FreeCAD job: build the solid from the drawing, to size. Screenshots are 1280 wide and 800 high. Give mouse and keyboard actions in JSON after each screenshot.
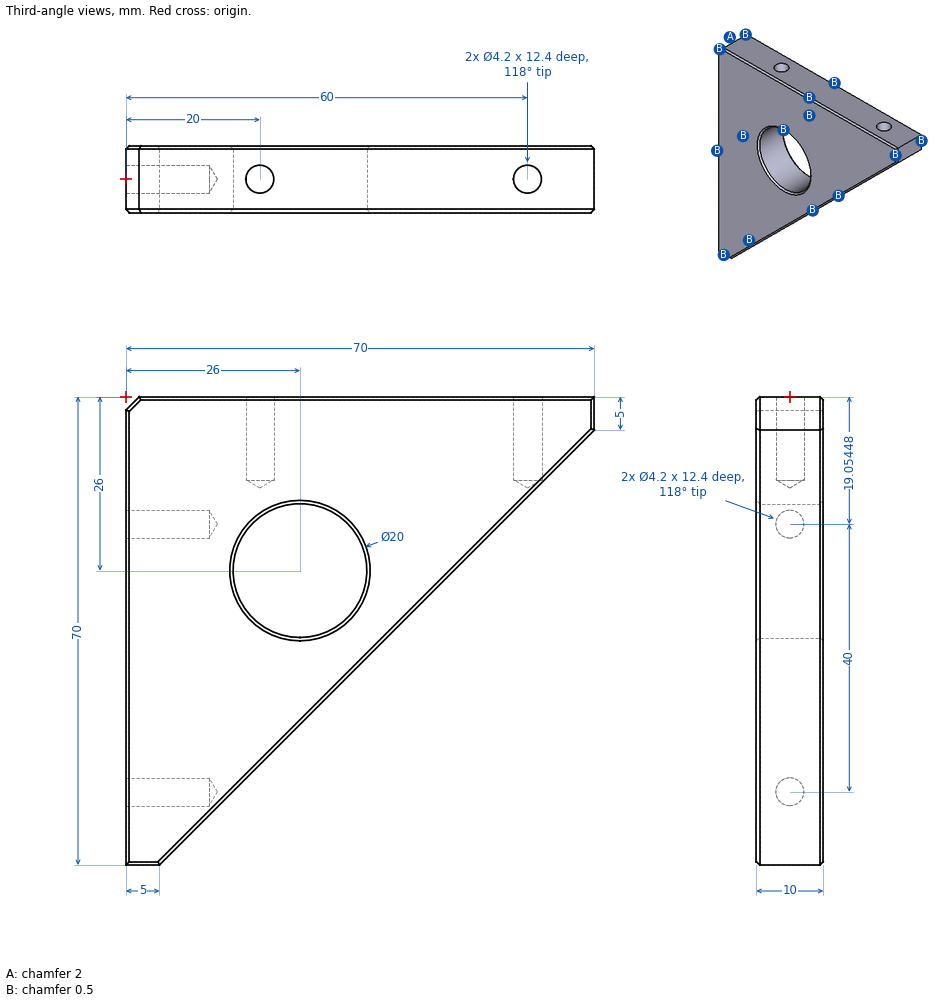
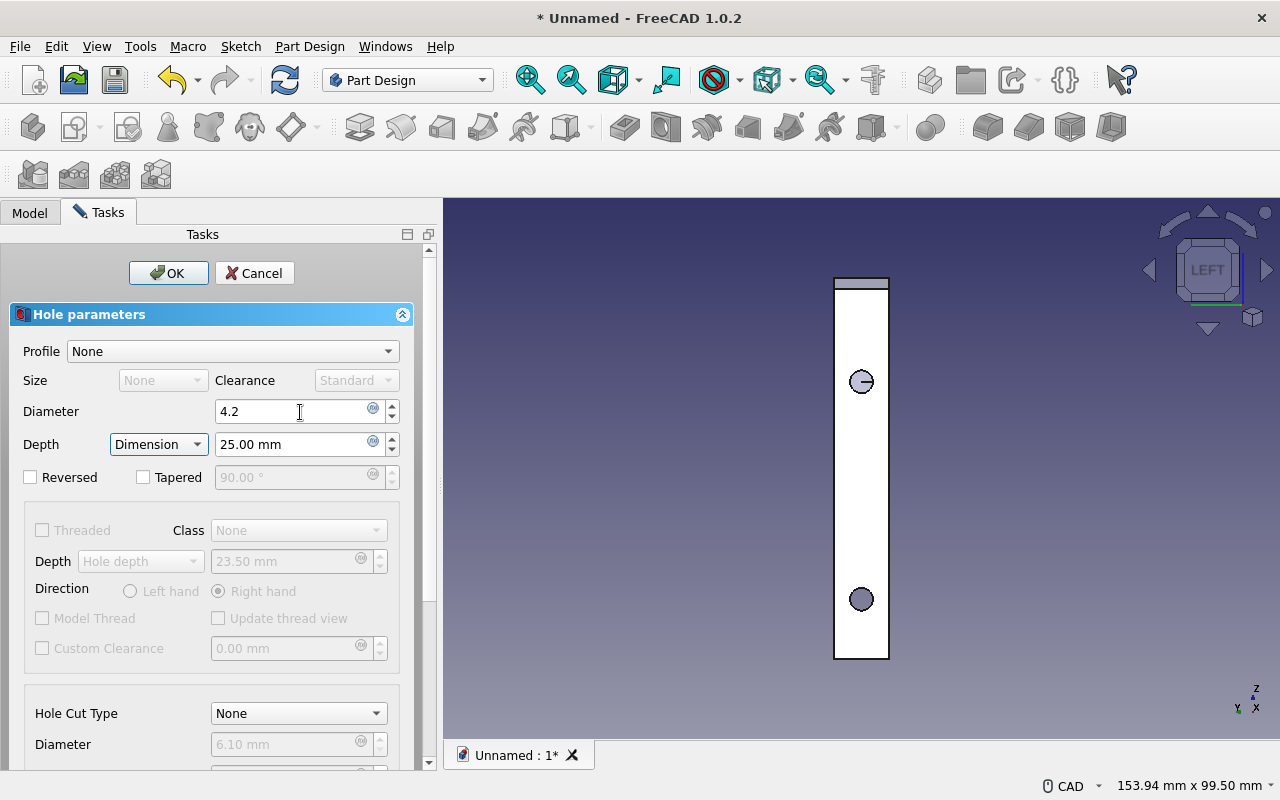
{"action": "triple_click", "coordinate": [300, 444]}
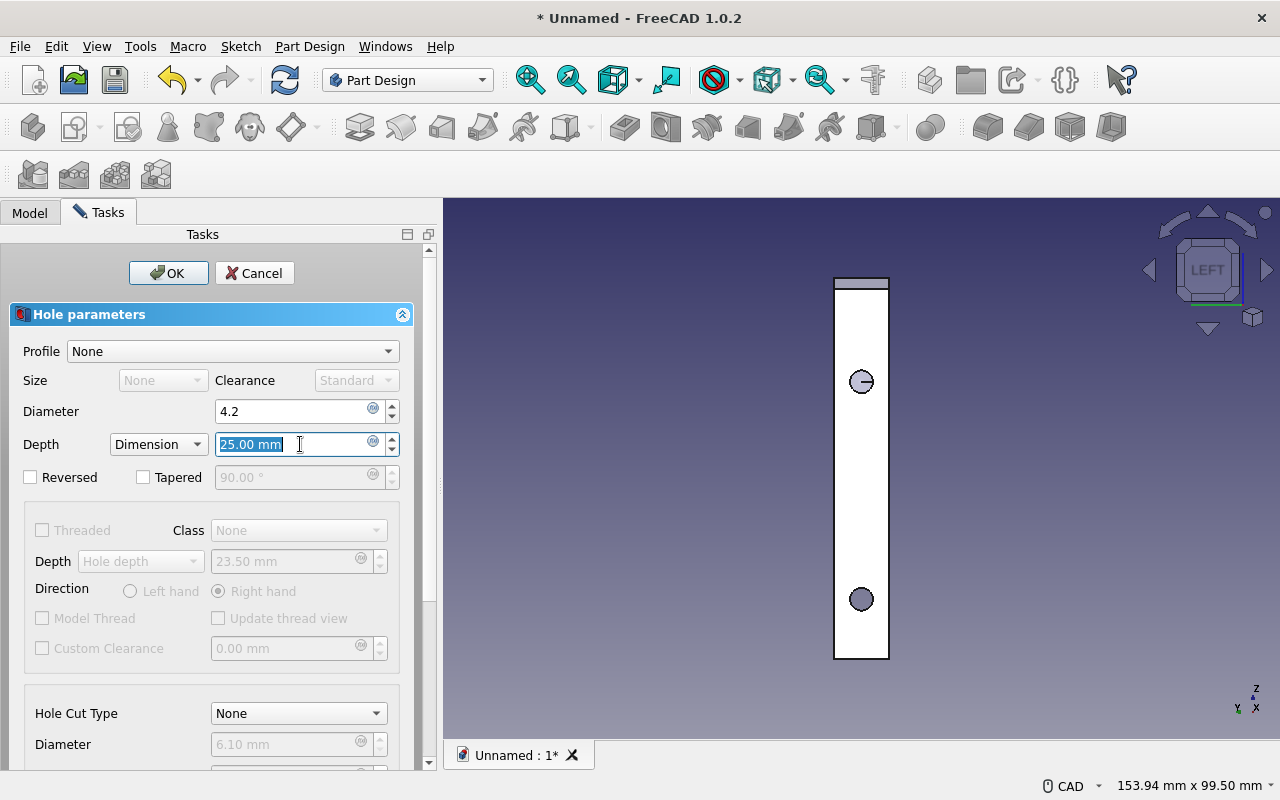
{"action": "type", "text": "12.4"}
{"action": "key", "text": "Tab"}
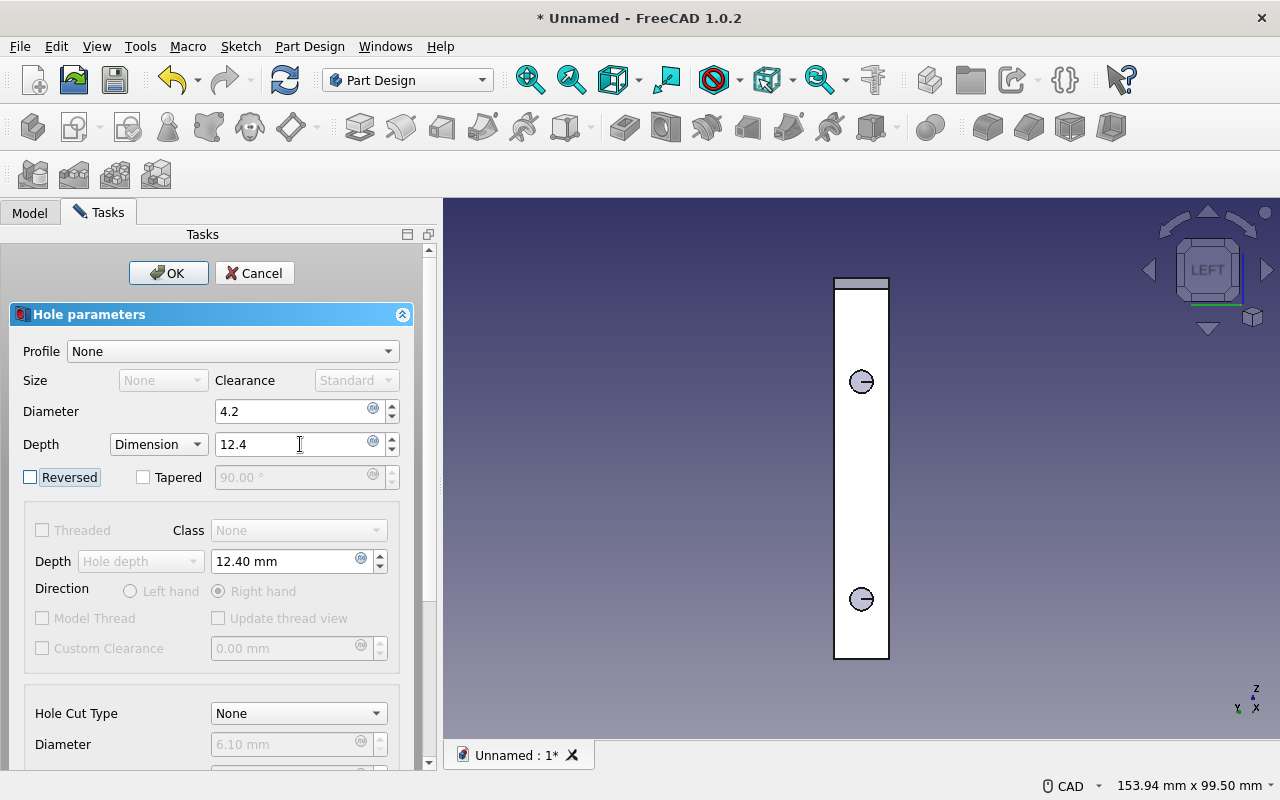
{"action": "left_click", "coordinate": [169, 273]}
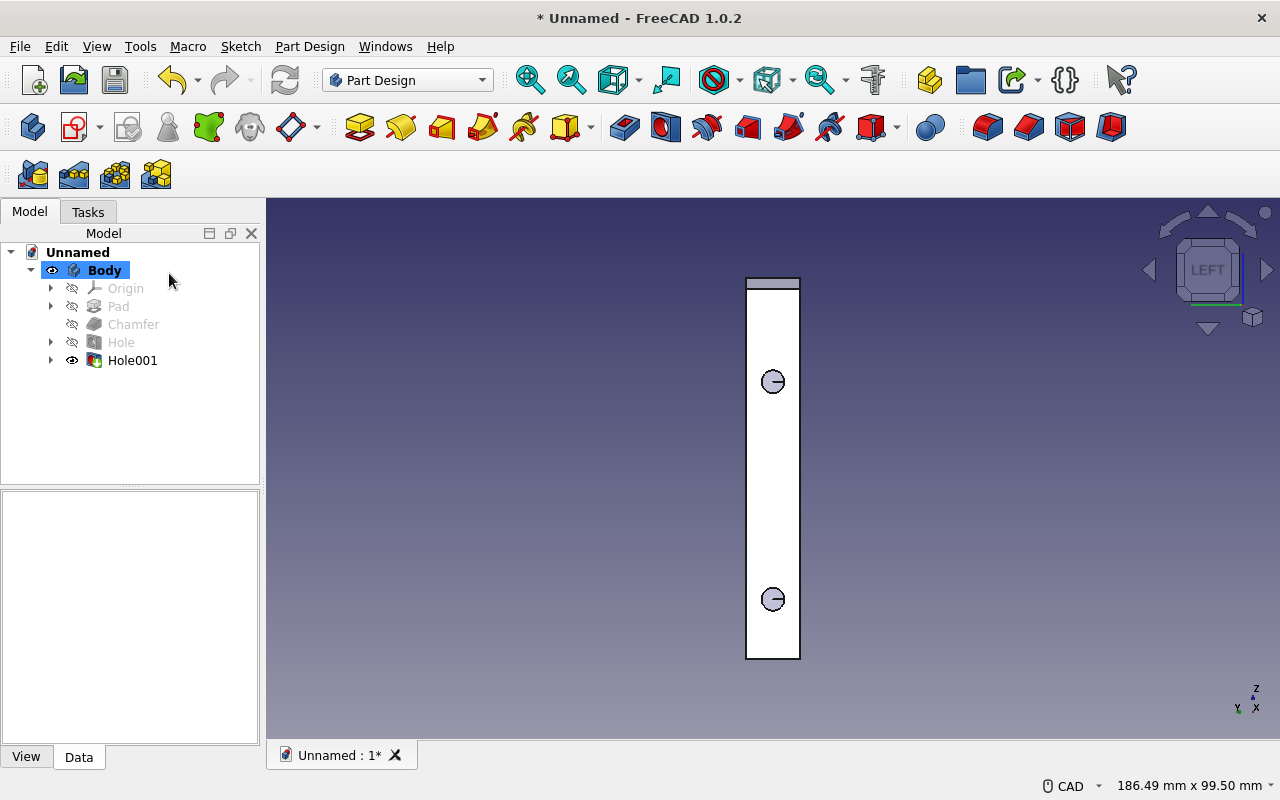
{"action": "key", "text": "0"}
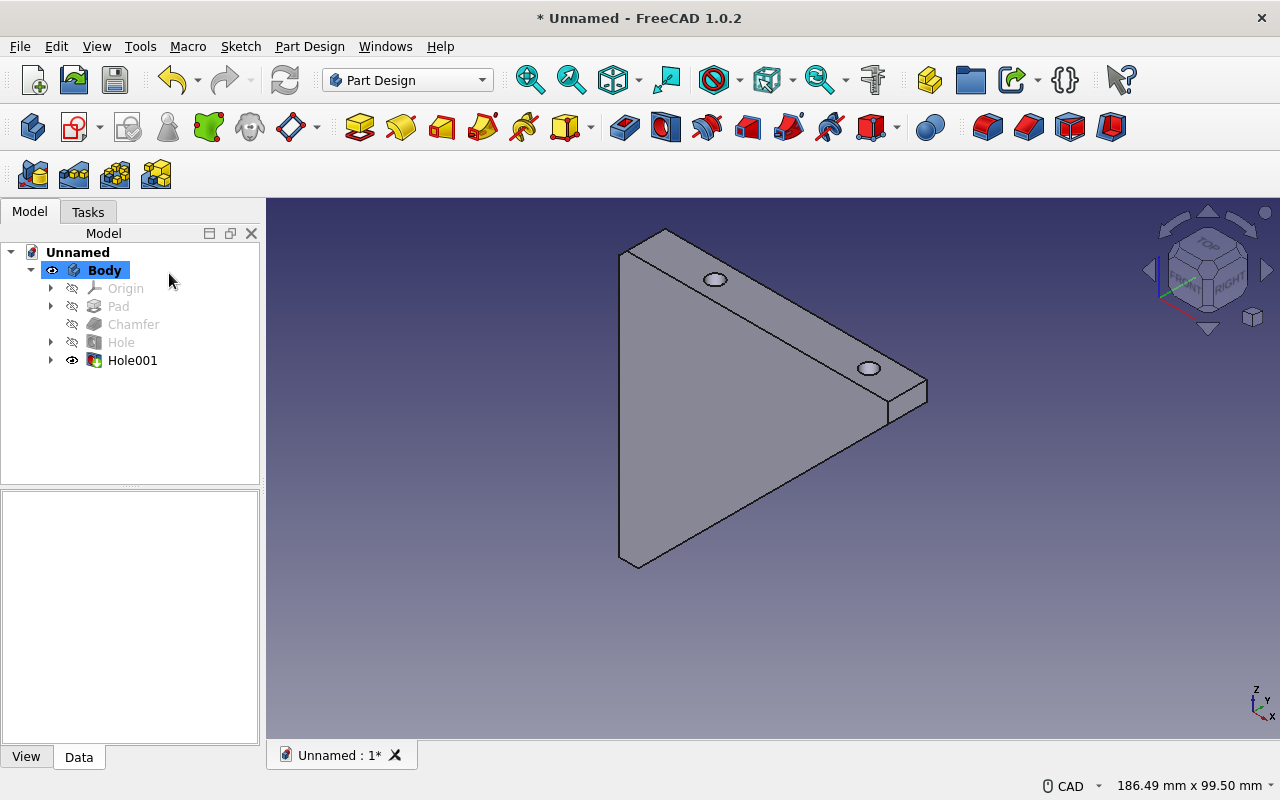
{"action": "left_click", "coordinate": [715, 412]}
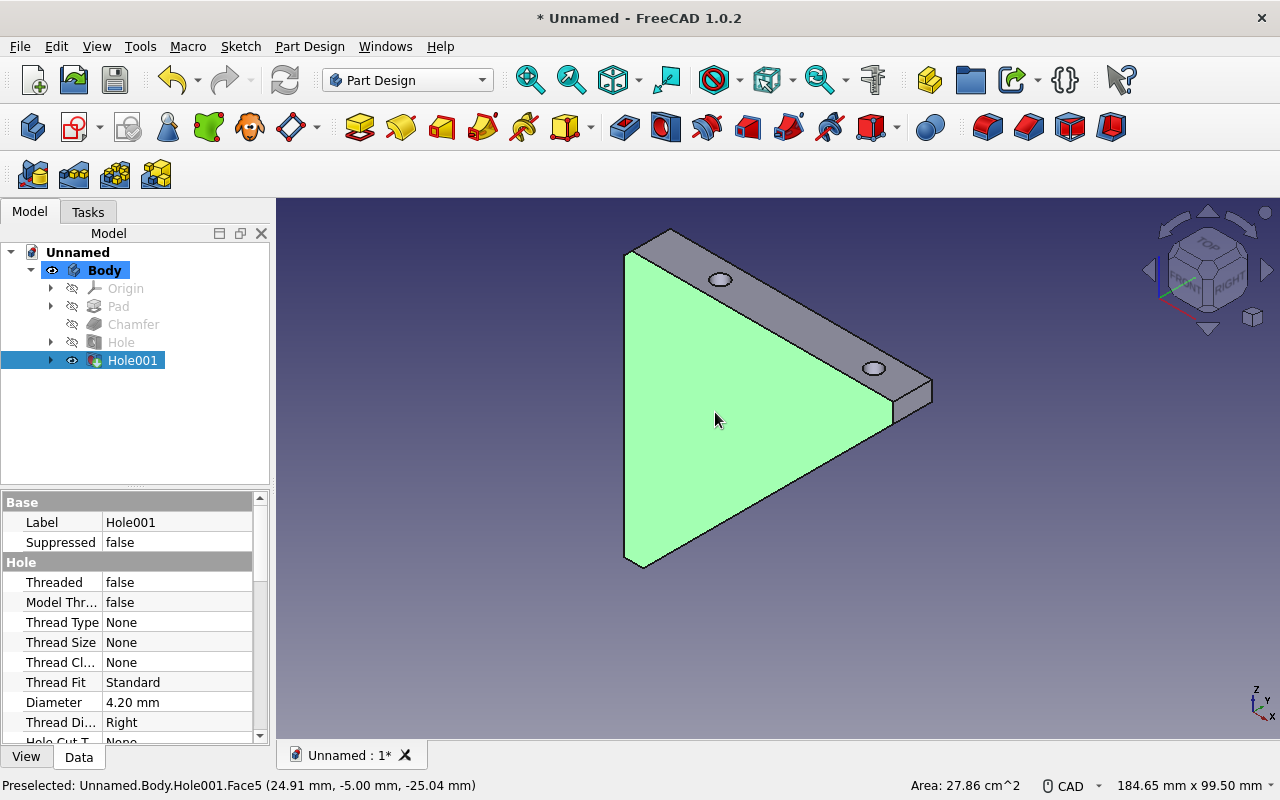
{"action": "left_click", "coordinate": [74, 128]}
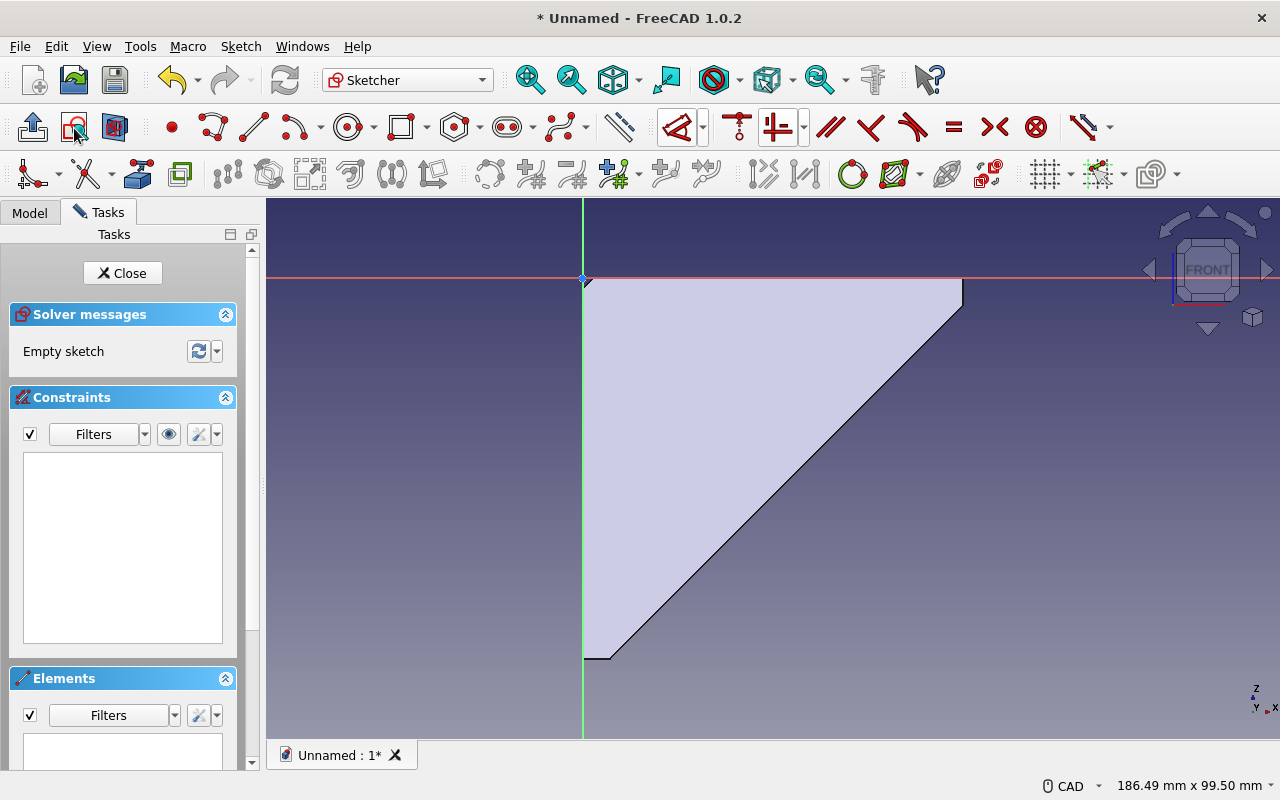
{"action": "scroll", "coordinate": [651, 264], "scroll_direction": "up", "scroll_amount": 3}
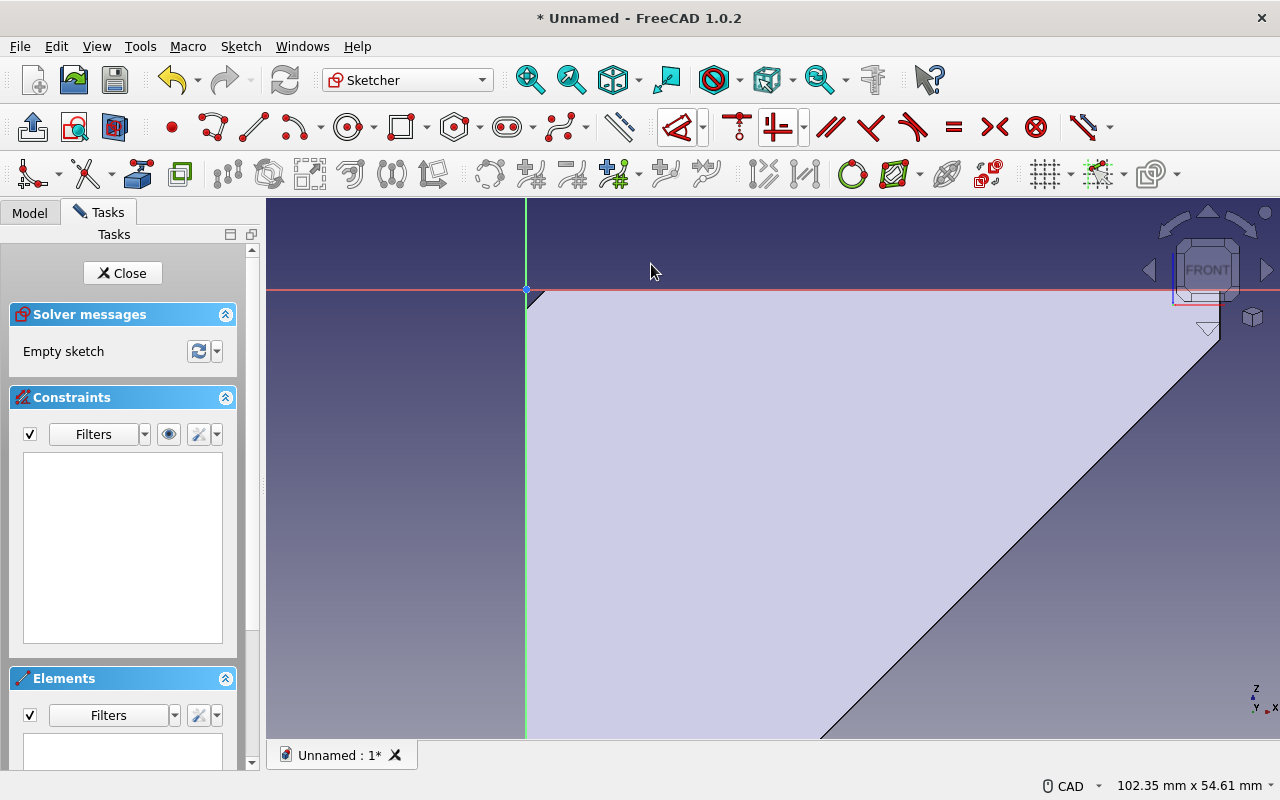
{"action": "left_click", "coordinate": [348, 128]}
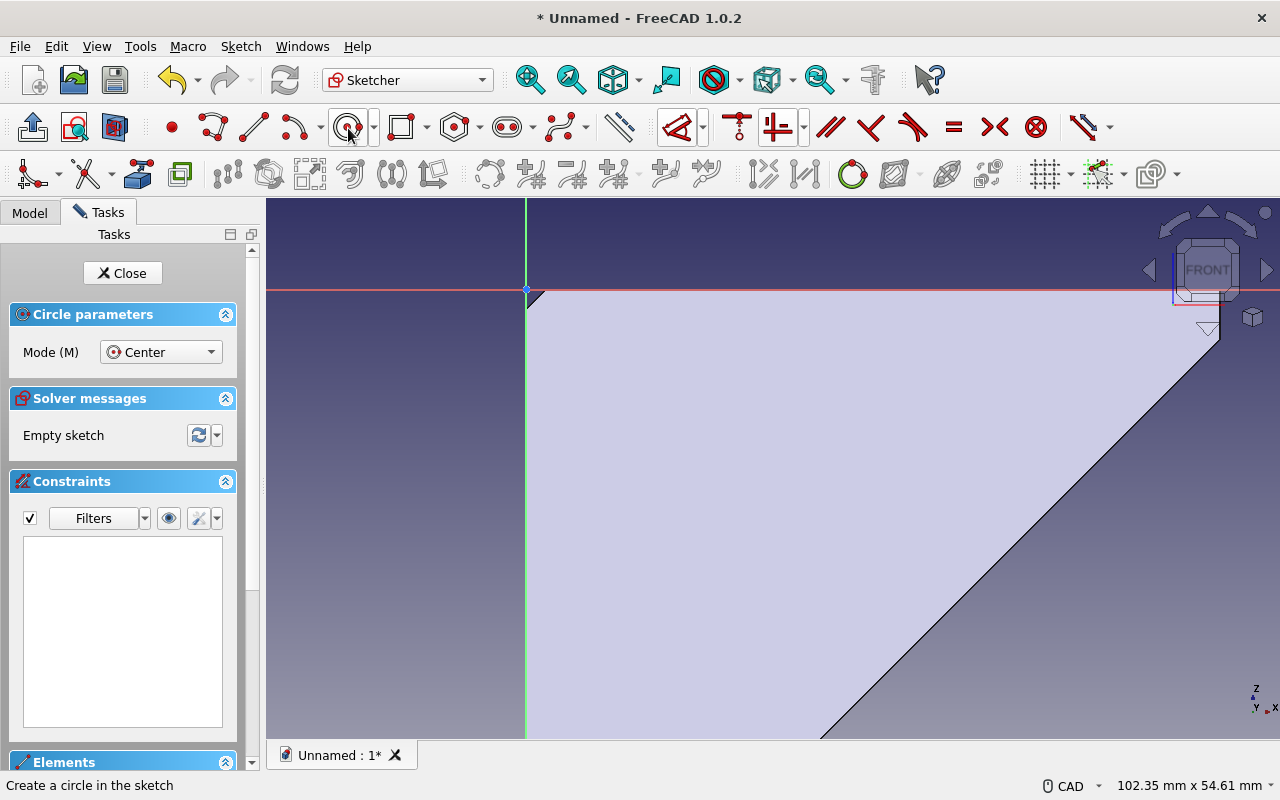
{"action": "left_click", "coordinate": [784, 547]}
{"action": "mouse_move", "coordinate": [854, 477]}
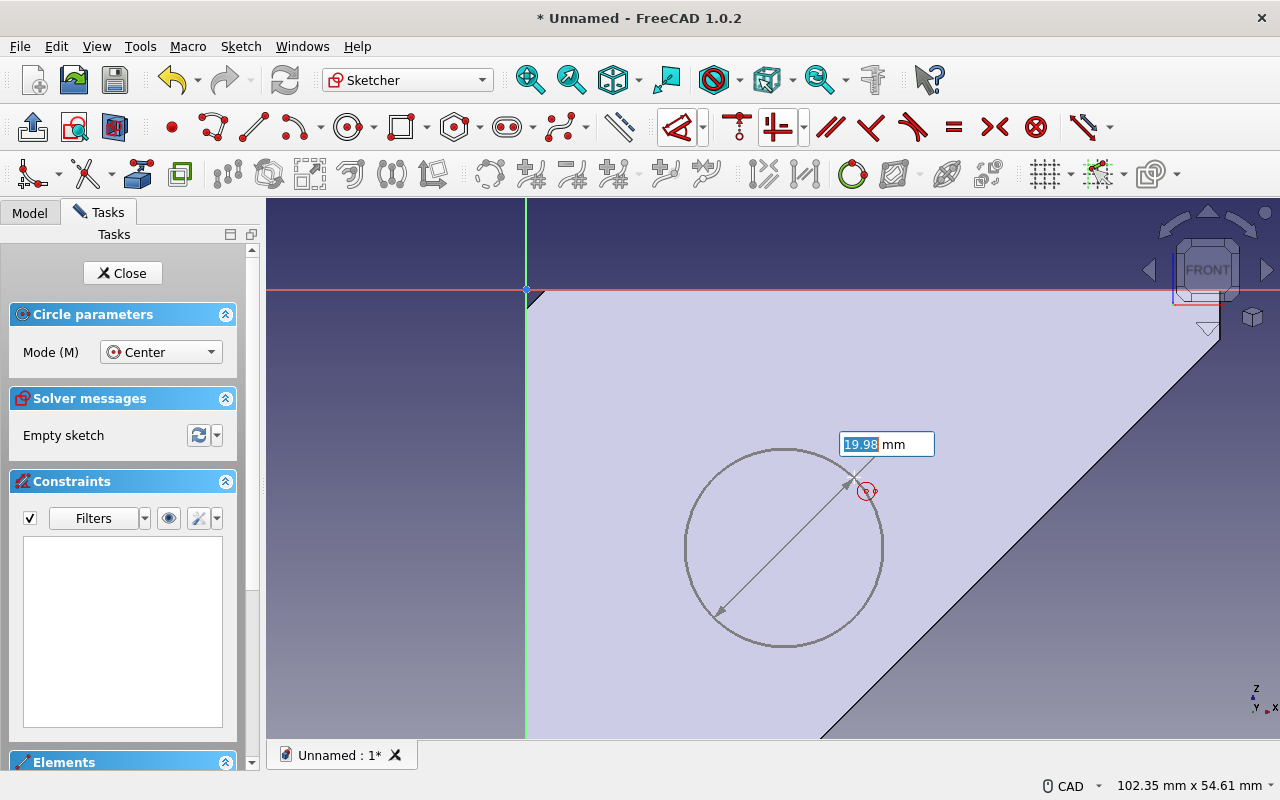
{"action": "type", "text": "20"}
{"action": "key", "text": "Return"}
{"action": "key", "text": "Escape"}